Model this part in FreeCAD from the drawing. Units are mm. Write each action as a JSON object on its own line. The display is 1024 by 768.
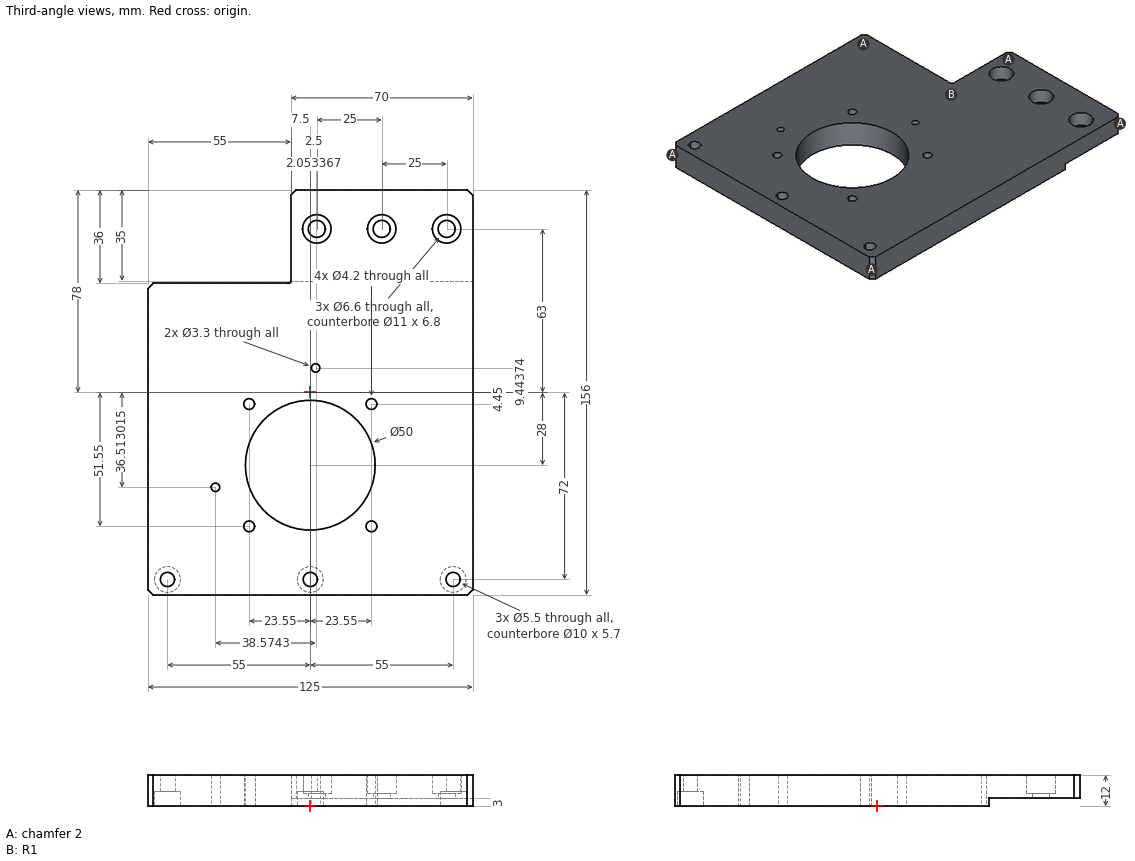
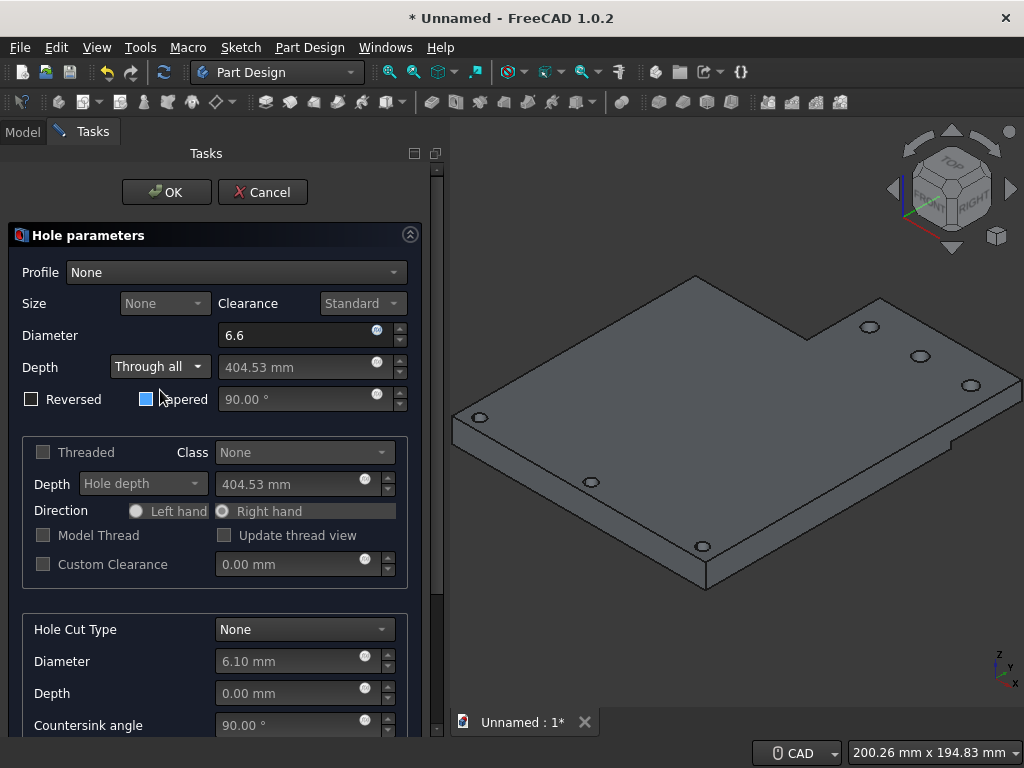
{"action": "left_click", "coordinate": [306, 630]}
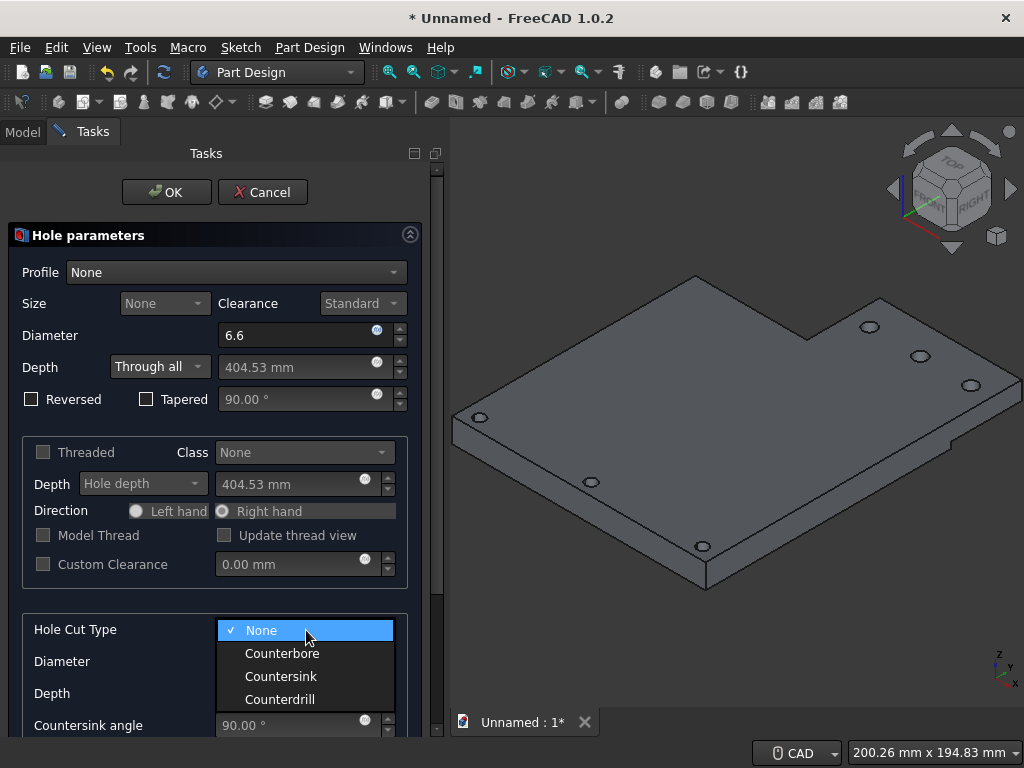
{"action": "left_click", "coordinate": [304, 654]}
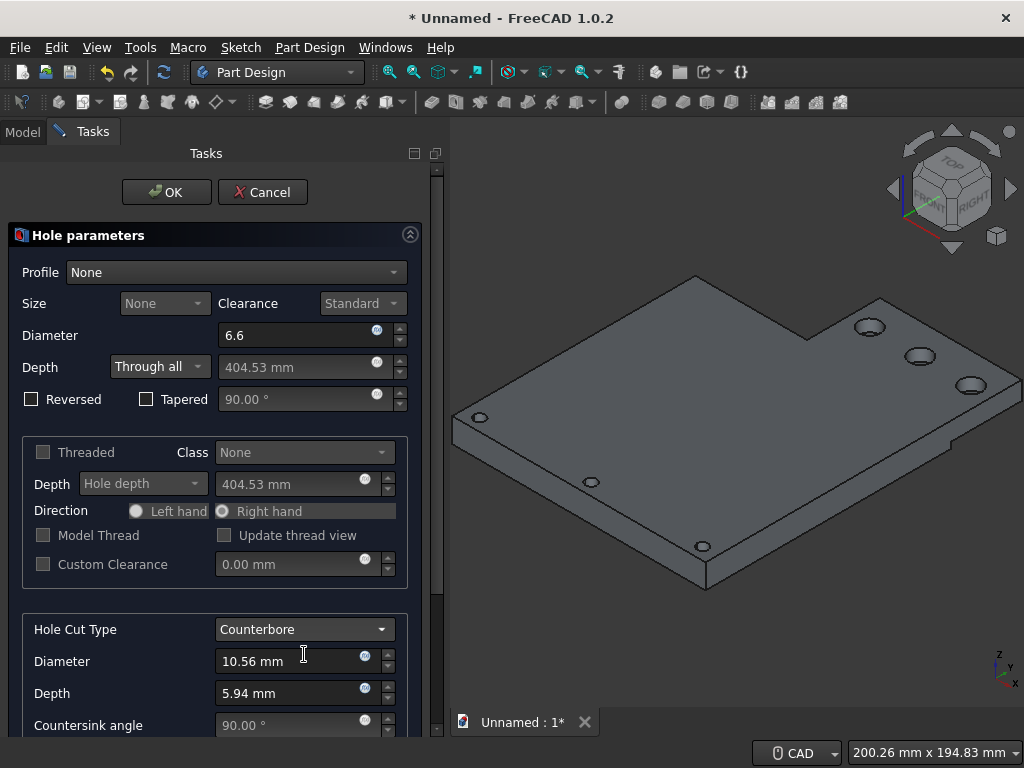
{"action": "triple_click", "coordinate": [298, 661]}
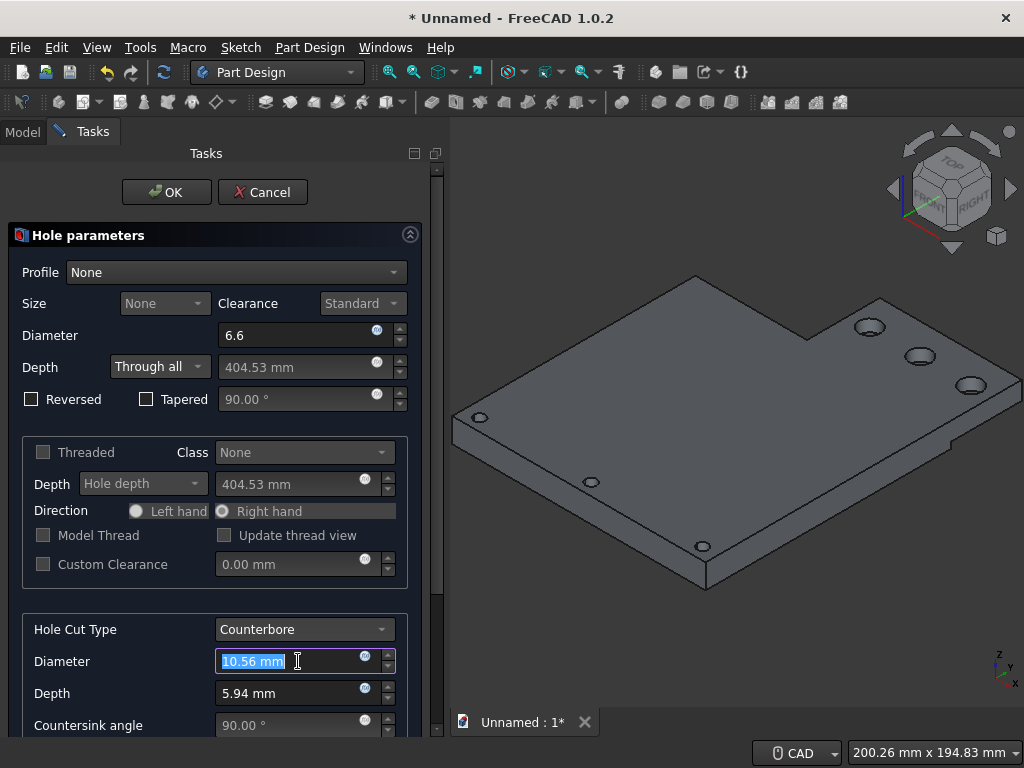
{"action": "type", "text": "11"}
{"action": "key", "text": "Tab"}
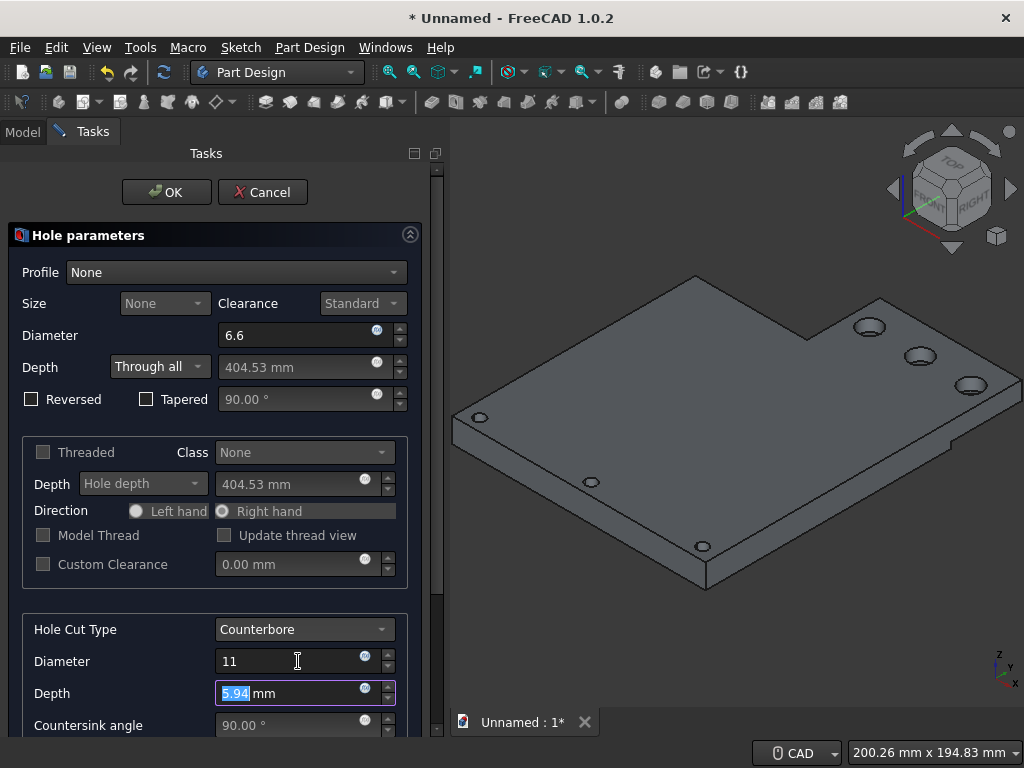
{"action": "type", "text": "6.8"}
{"action": "key", "text": "Tab"}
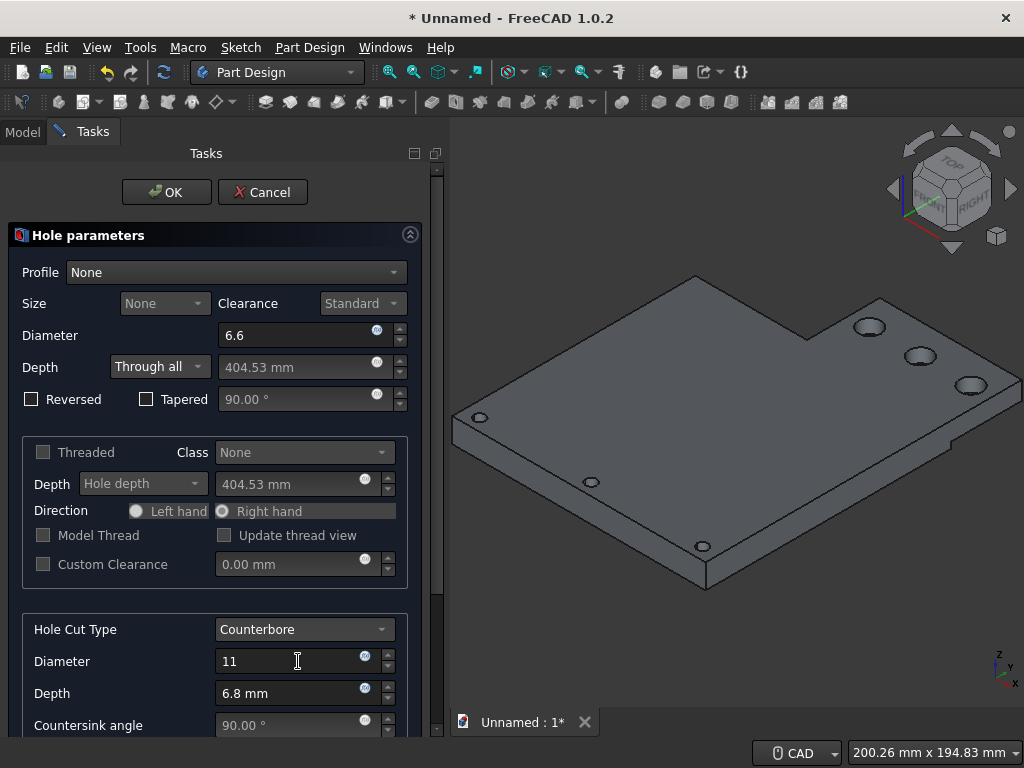
{"action": "left_click", "coordinate": [167, 192]}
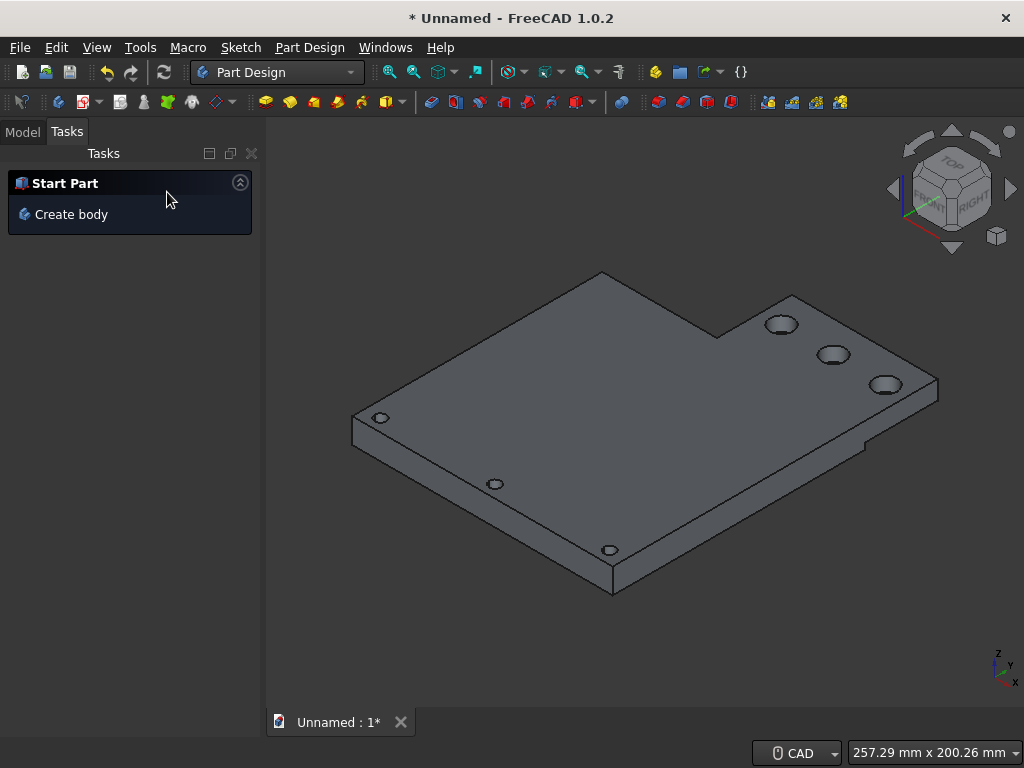
{"action": "left_click", "coordinate": [613, 580]}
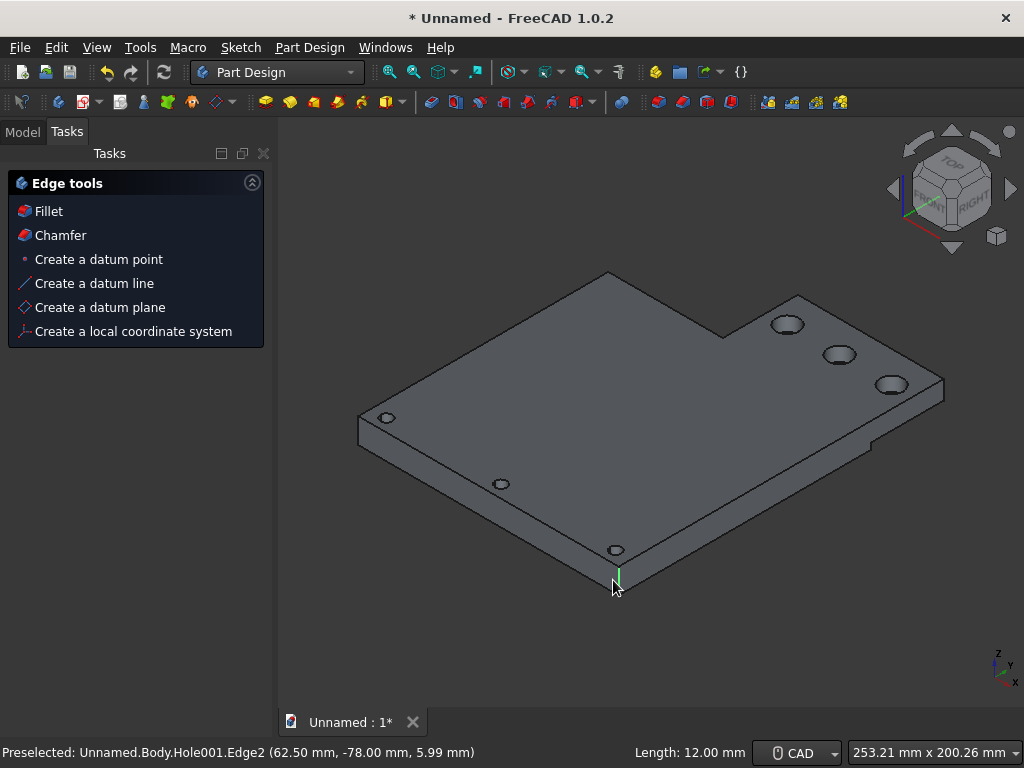
{"action": "key", "text": "2"}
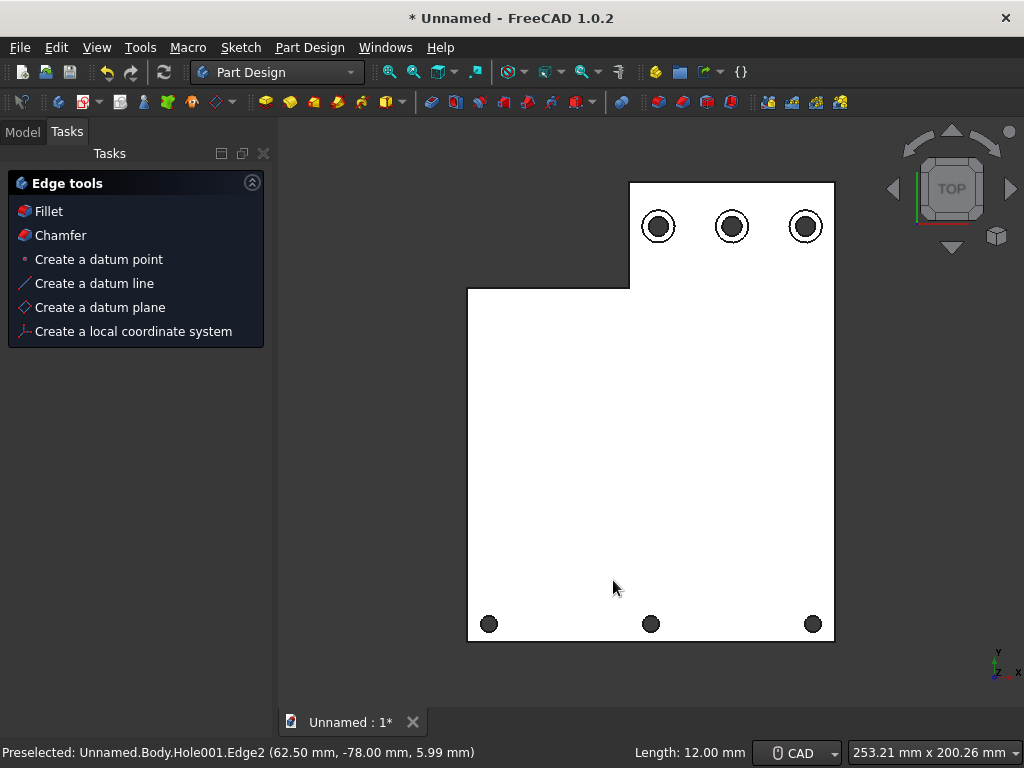
{"action": "key", "text": "0"}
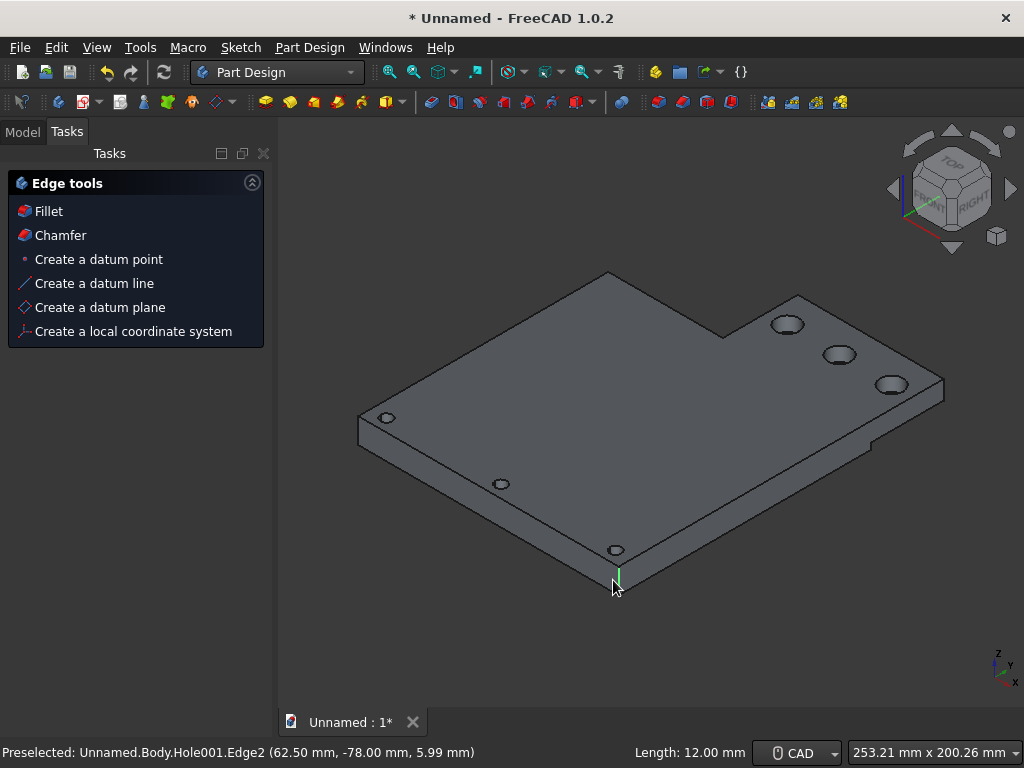
{"action": "key", "text": "1"}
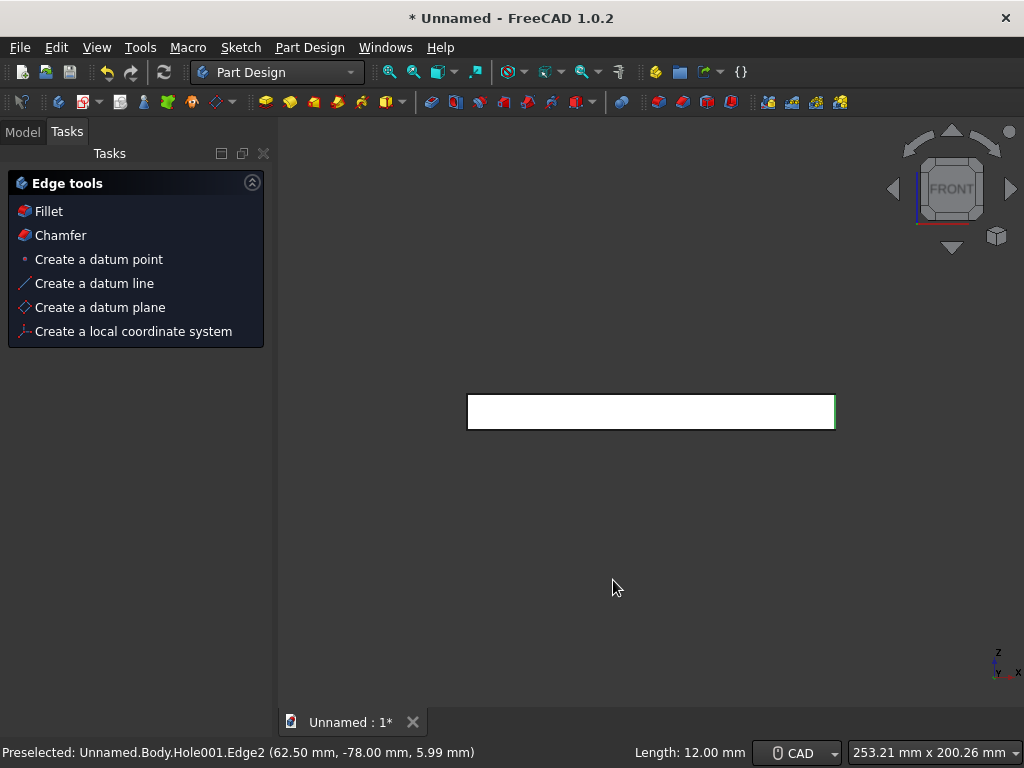
{"action": "left_click", "coordinate": [467, 411], "text": "ctrl"}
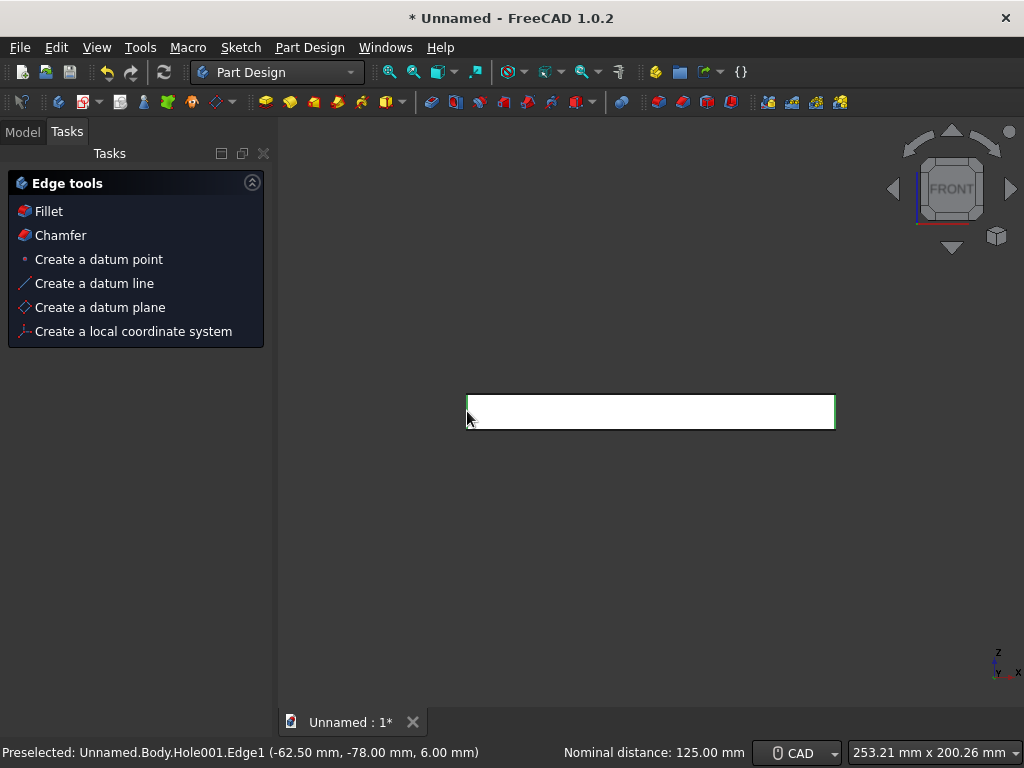
{"action": "key", "text": "3"}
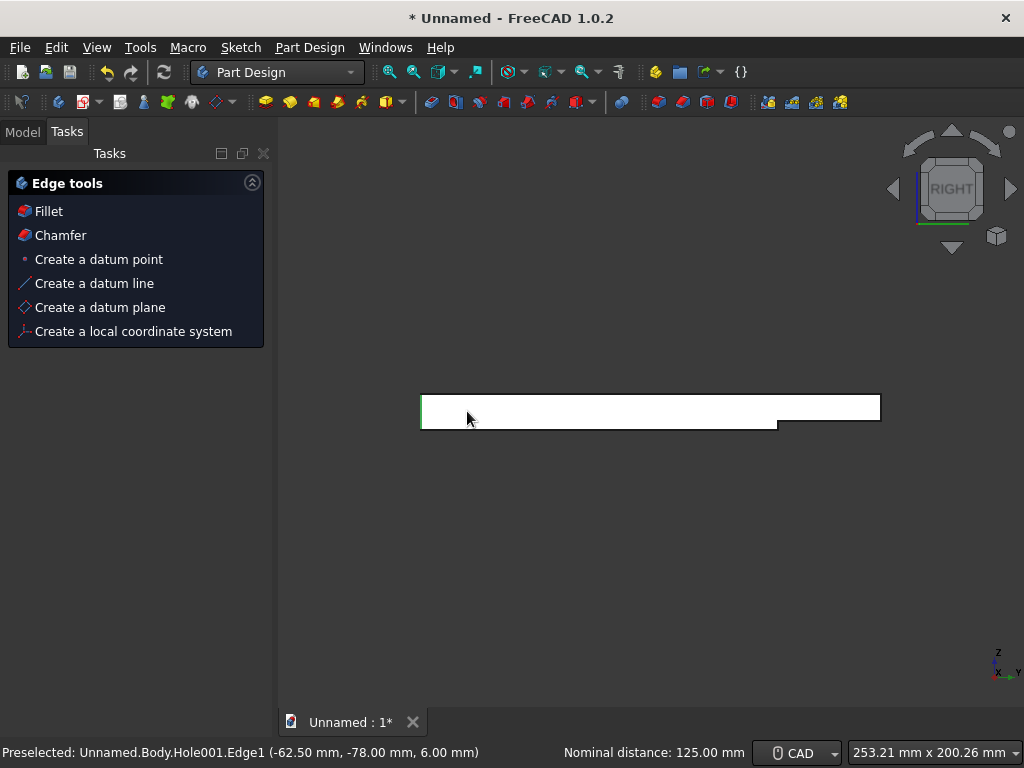
{"action": "left_click", "coordinate": [881, 407], "text": "ctrl"}